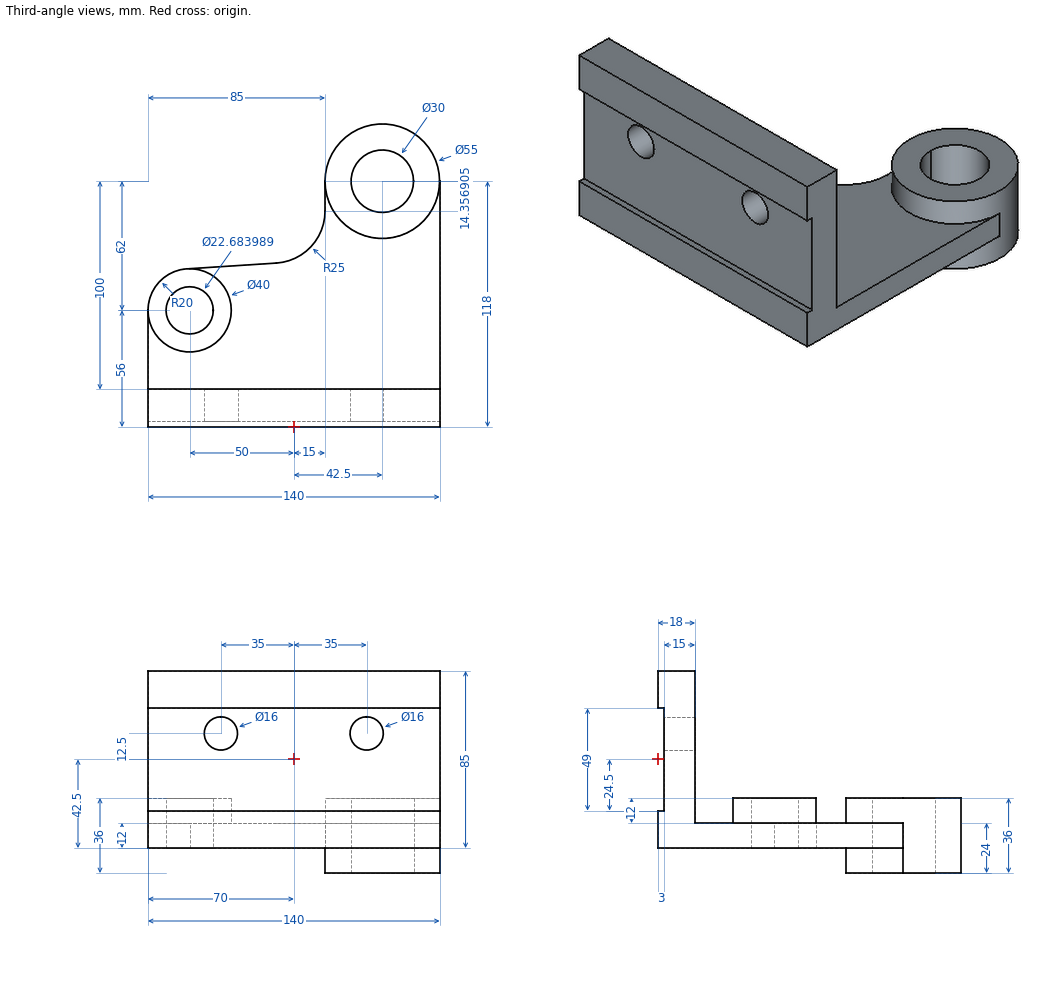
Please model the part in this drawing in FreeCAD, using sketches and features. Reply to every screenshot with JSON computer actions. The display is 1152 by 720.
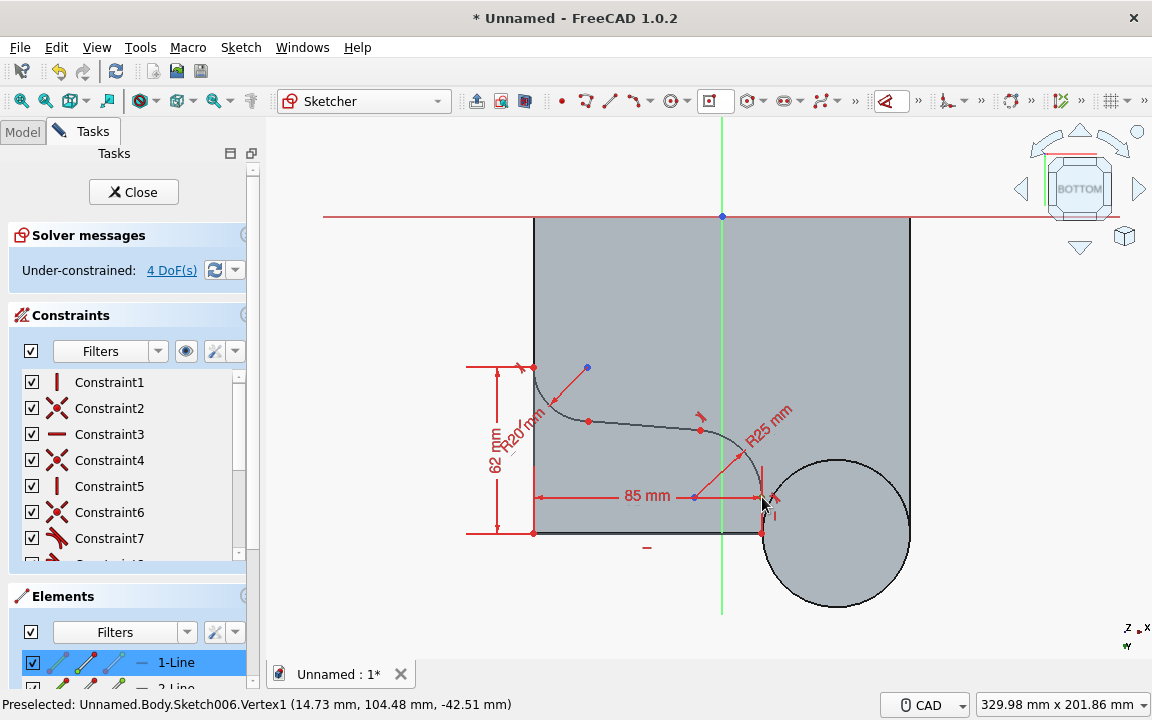
{"action": "key", "text": "l"}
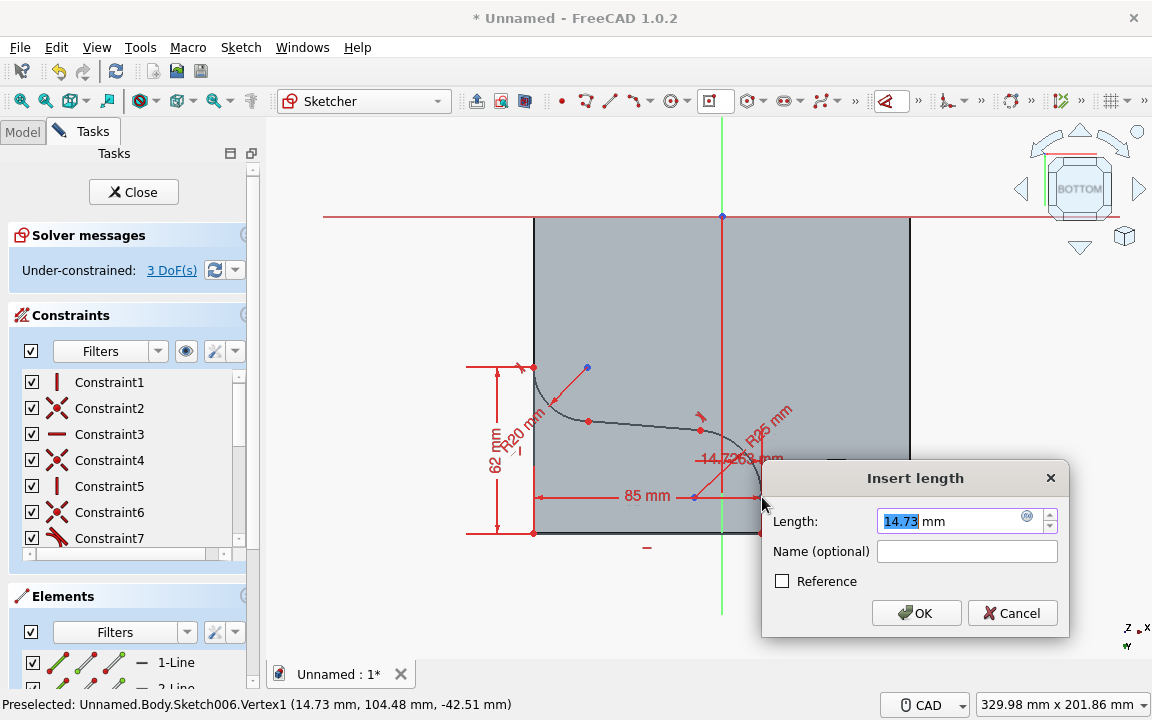
{"action": "type", "text": "15"}
{"action": "key", "text": "Return"}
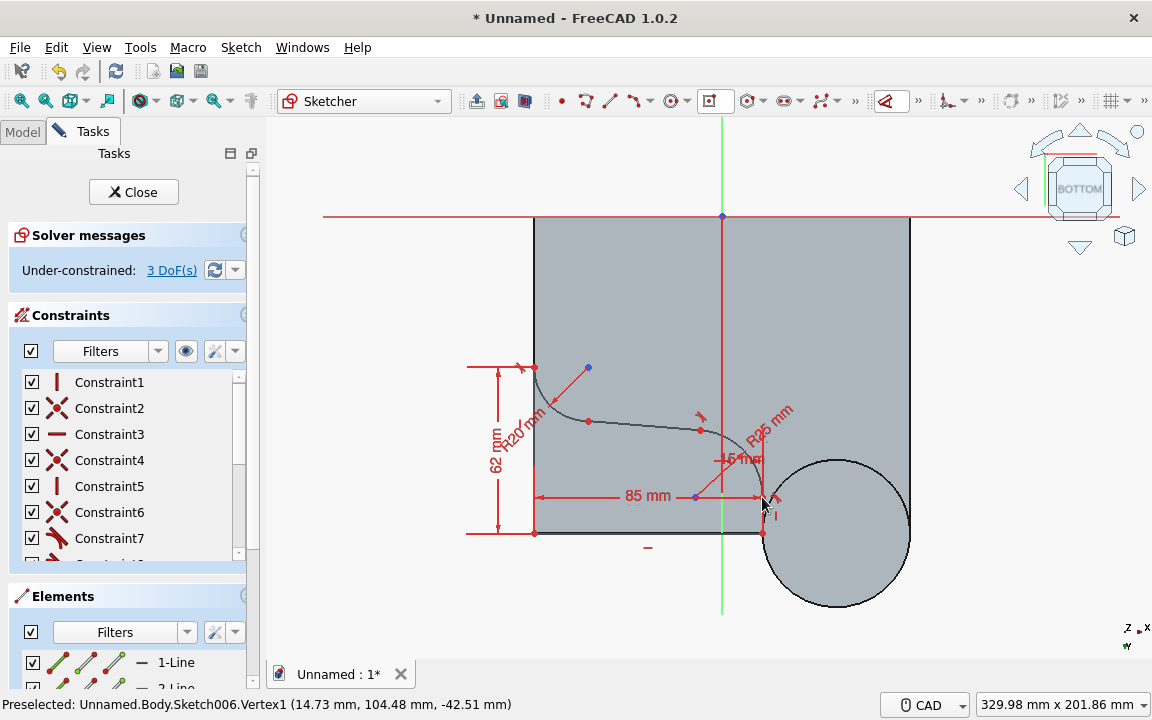
{"action": "left_click", "coordinate": [534, 367]}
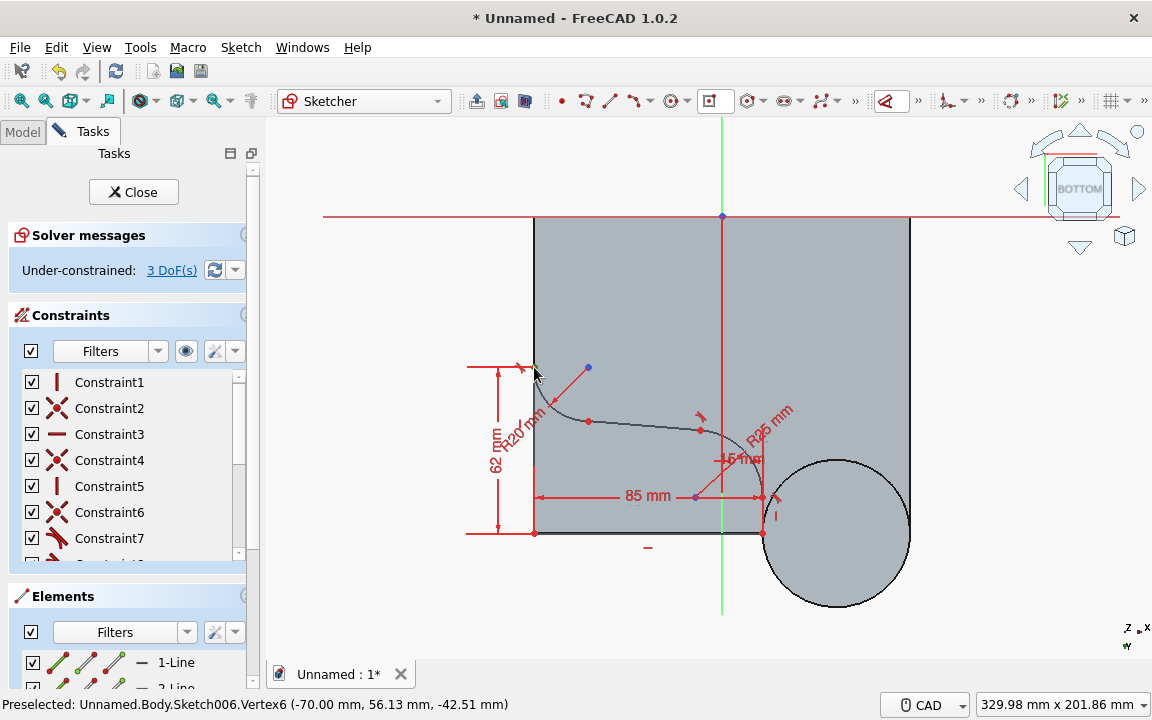
{"action": "left_click", "coordinate": [904, 102]}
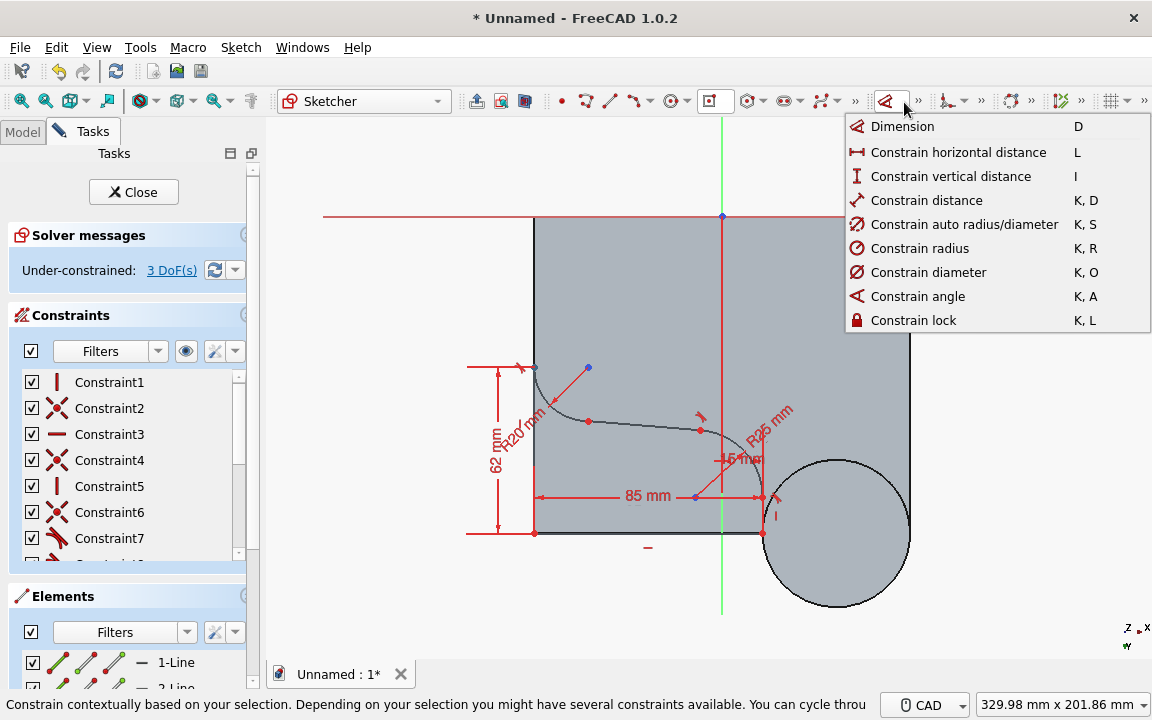
{"action": "left_click", "coordinate": [998, 176]}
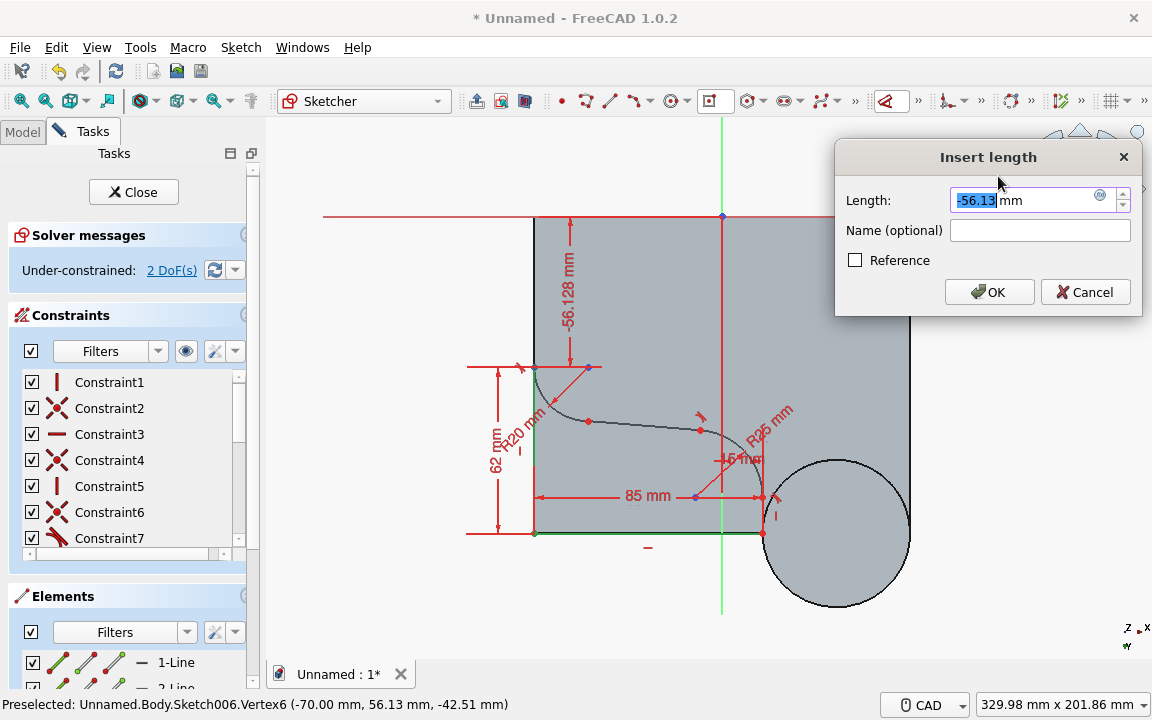
{"action": "type", "text": "-56"}
{"action": "key", "text": "Return"}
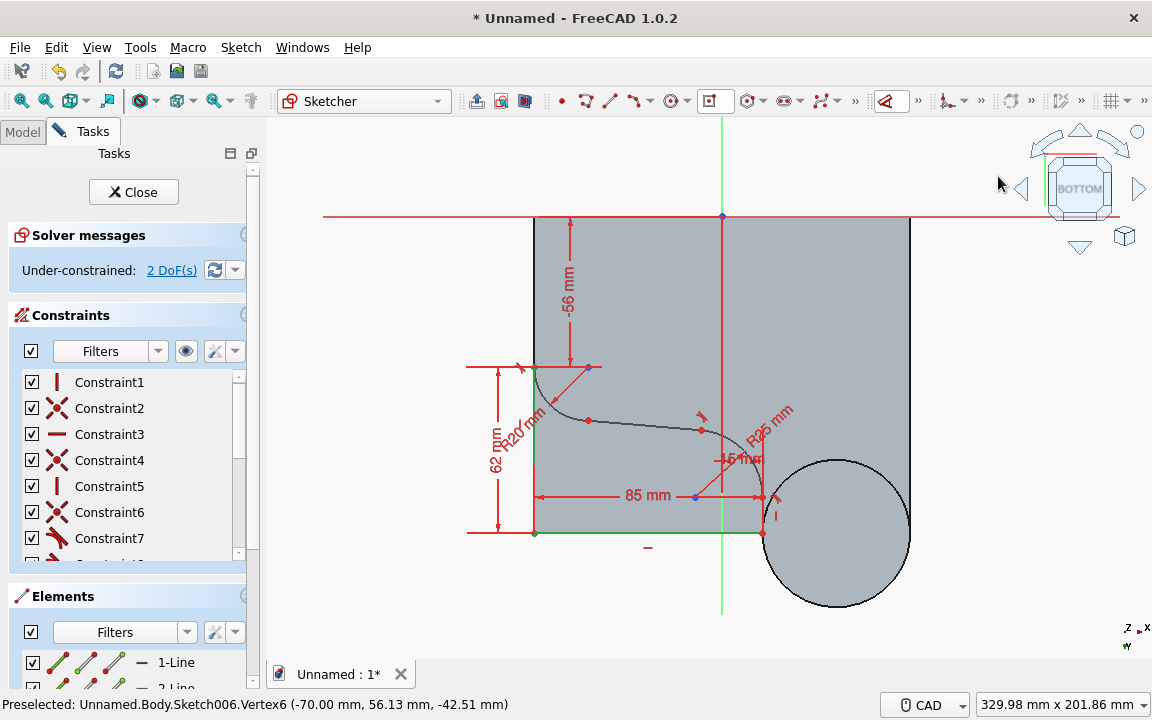
{"action": "left_click", "coordinate": [588, 421]}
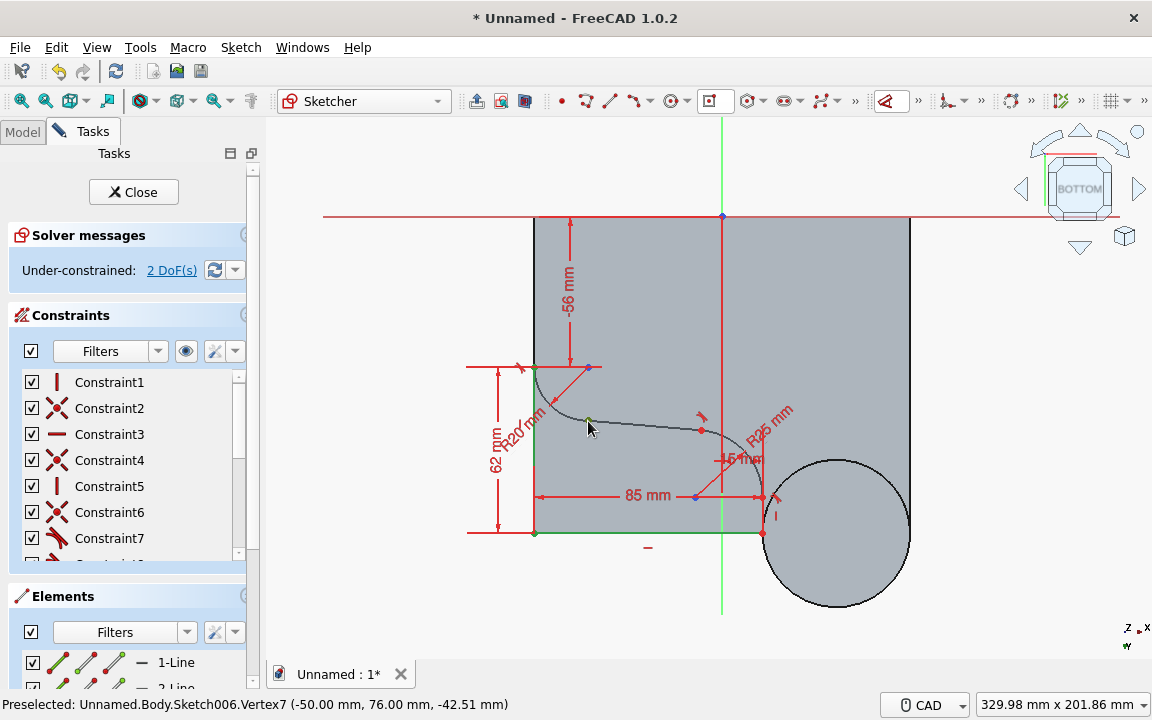
{"action": "key", "text": "l"}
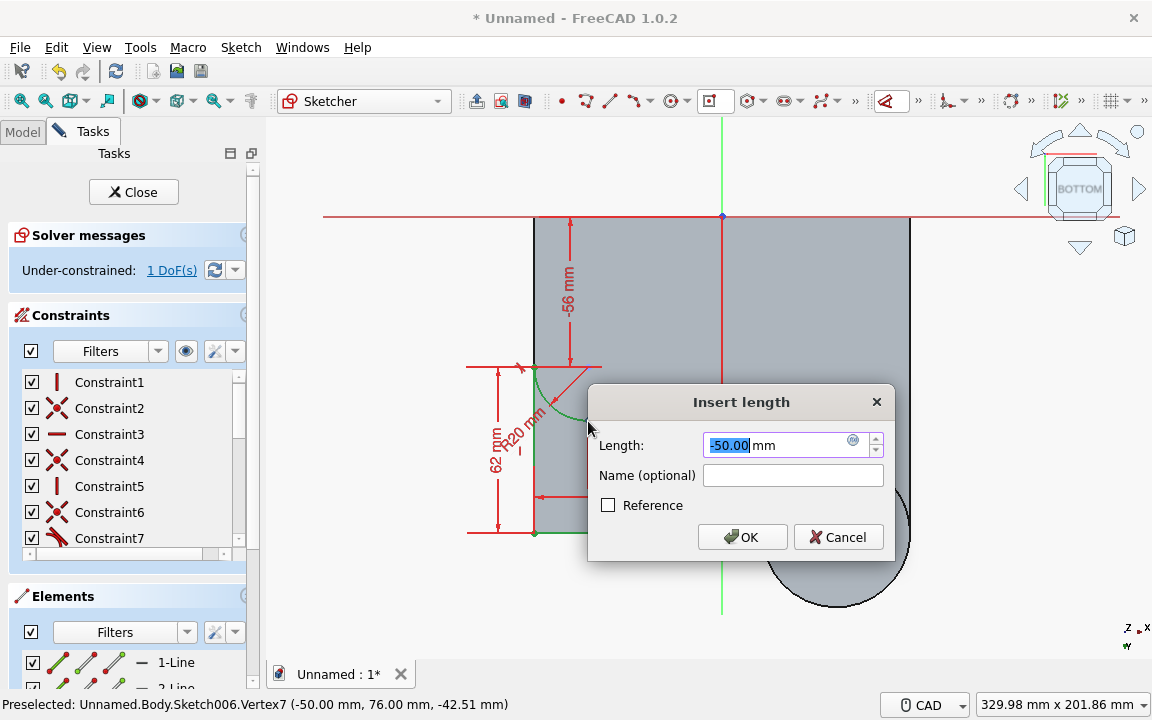
{"action": "type", "text": "-50"}
{"action": "key", "text": "Return"}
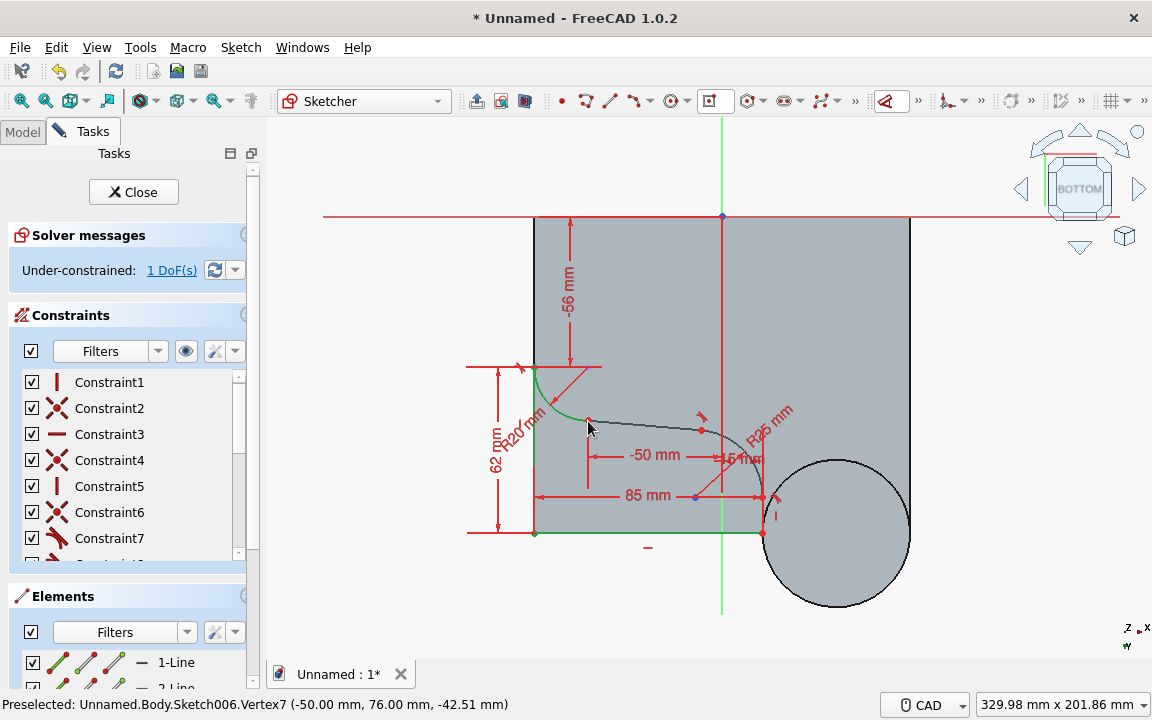
{"action": "scroll", "coordinate": [763, 508], "scroll_direction": "up", "scroll_amount": 2}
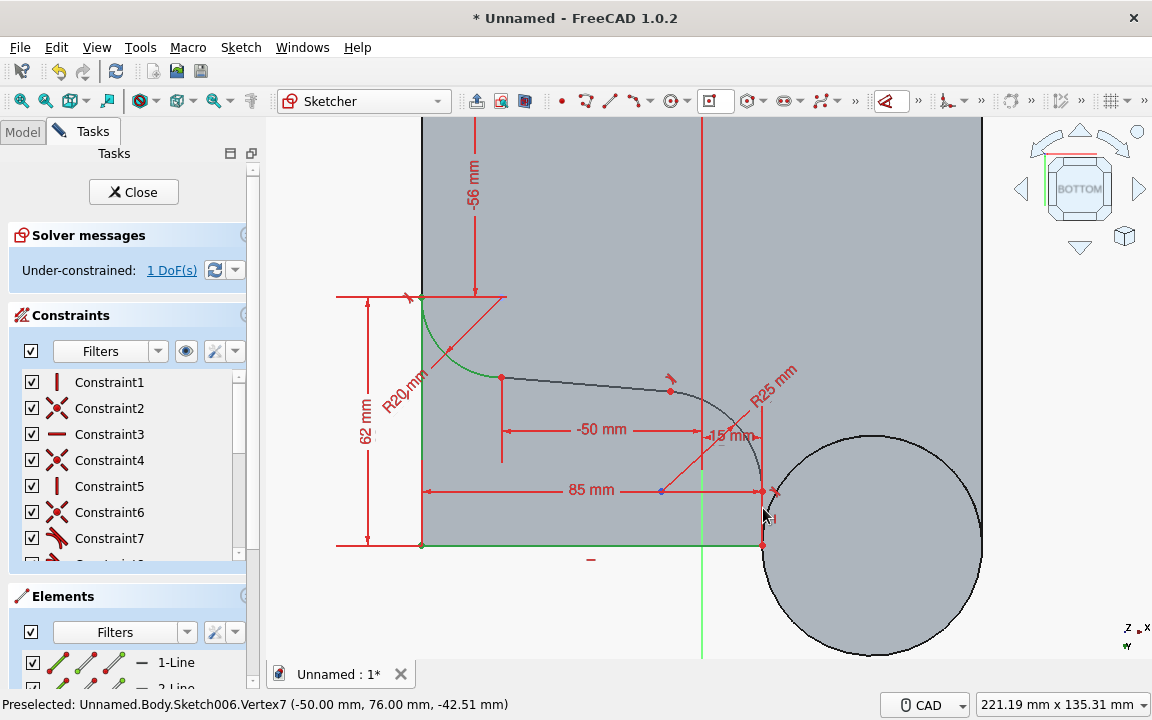
{"action": "left_click", "coordinate": [762, 508]}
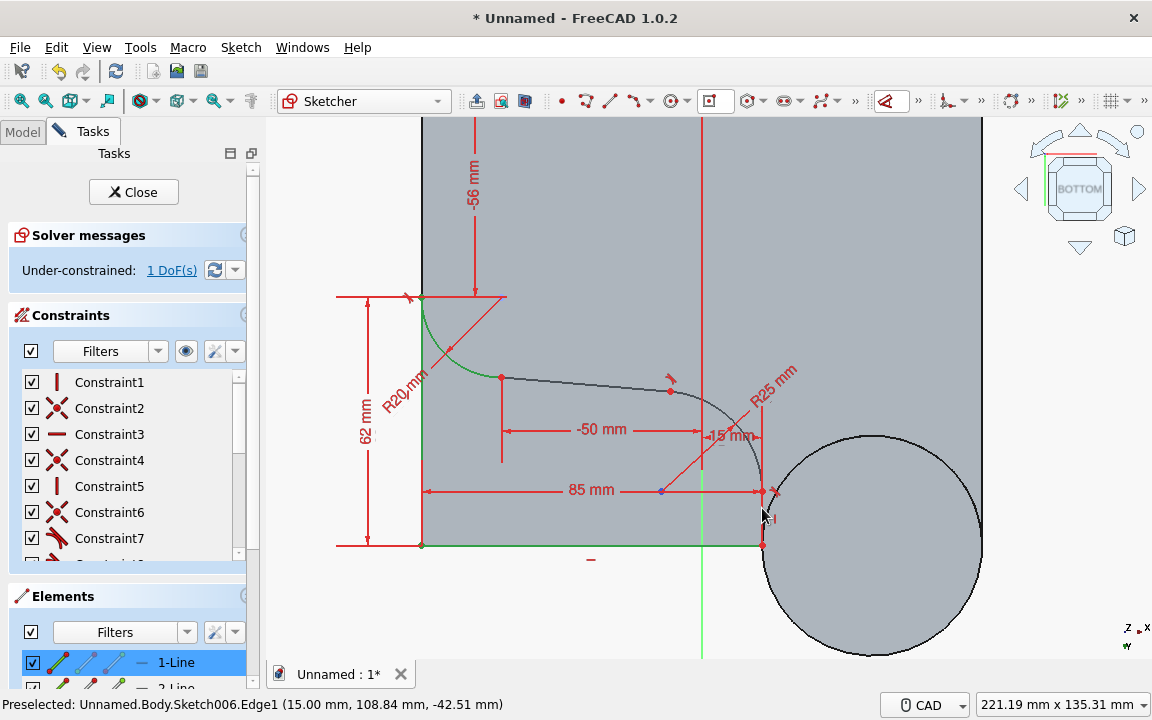
{"action": "key", "text": "i"}